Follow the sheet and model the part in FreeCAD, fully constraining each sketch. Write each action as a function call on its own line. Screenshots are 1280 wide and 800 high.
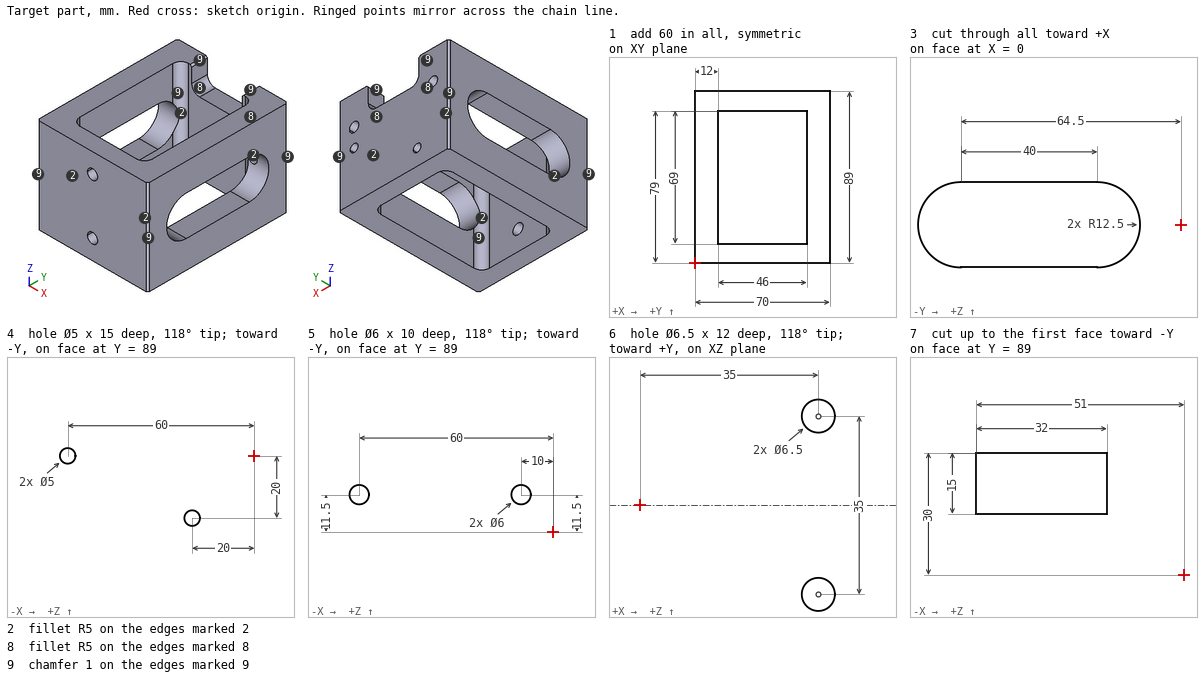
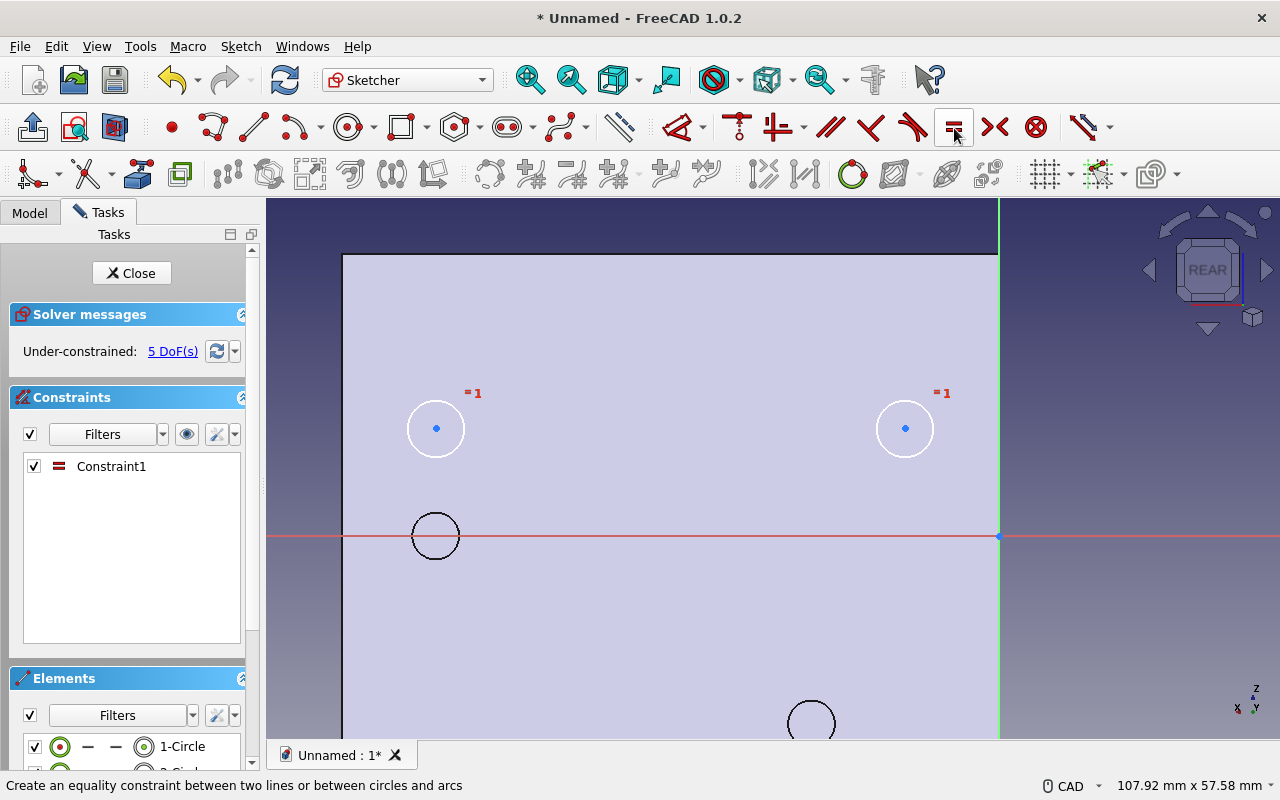
click(925, 409)
click(948, 386)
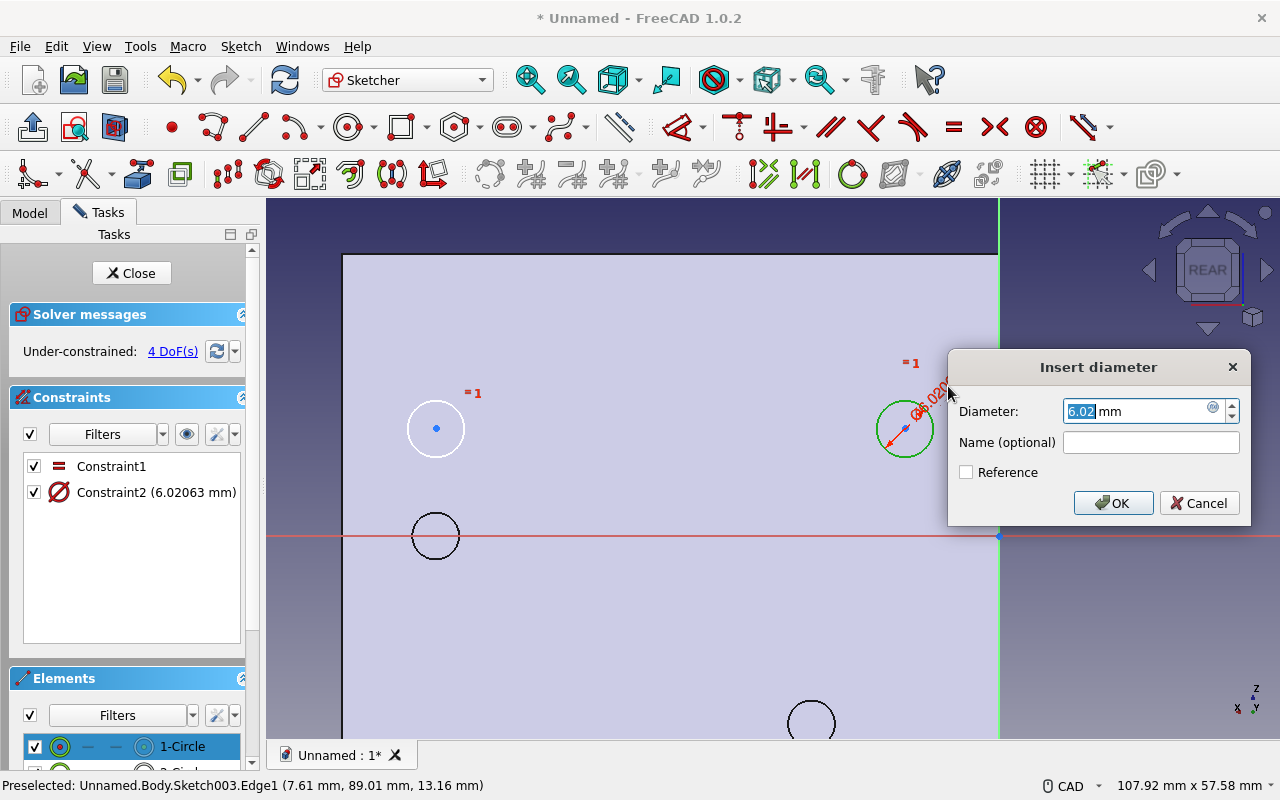
text(6)
key(Return)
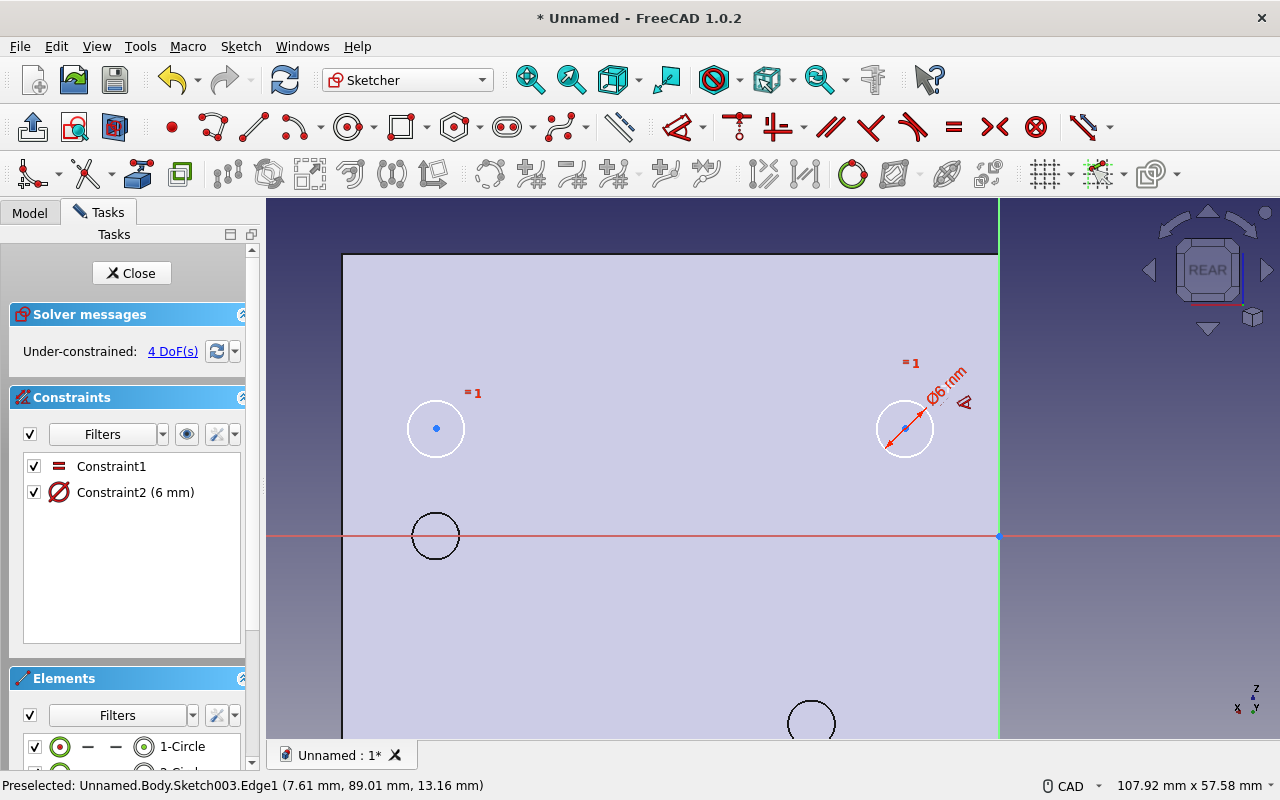
click(905, 429)
click(952, 570)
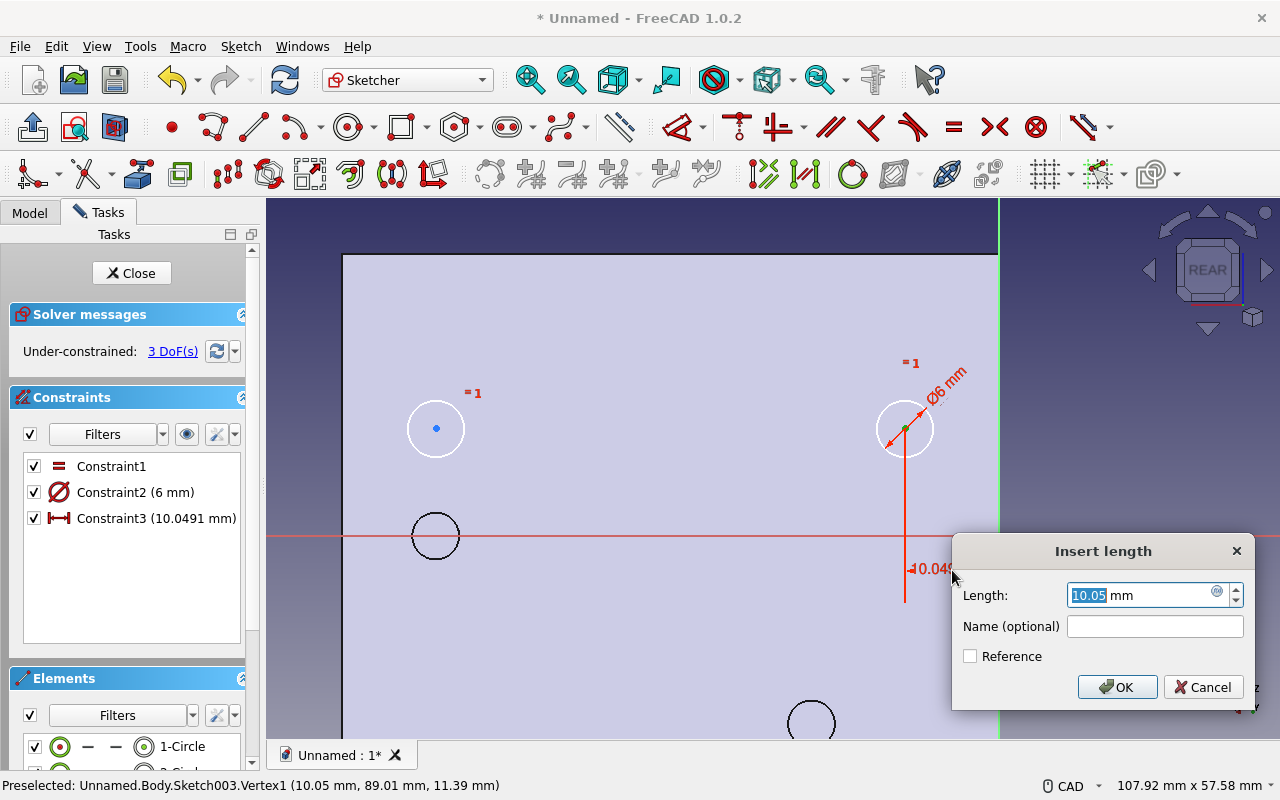
text(10)
key(Return)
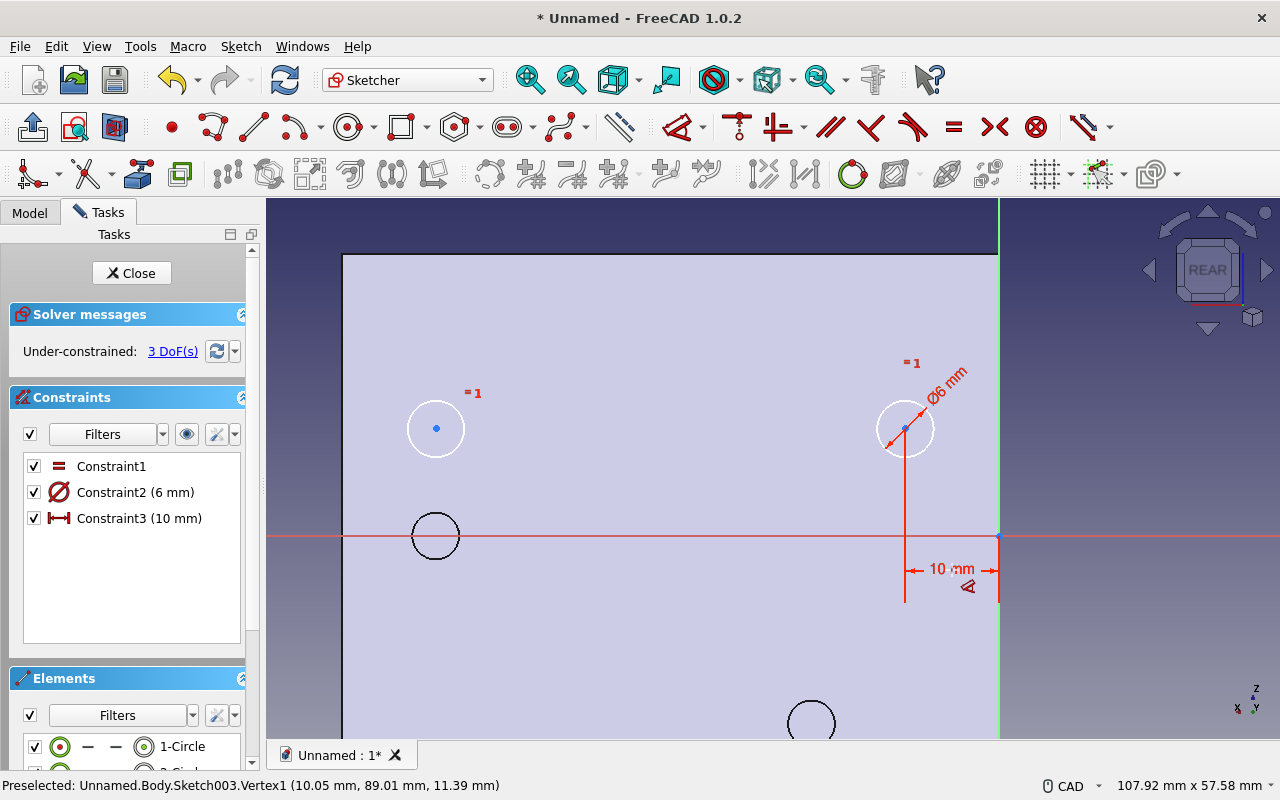
click(436, 429)
click(718, 570)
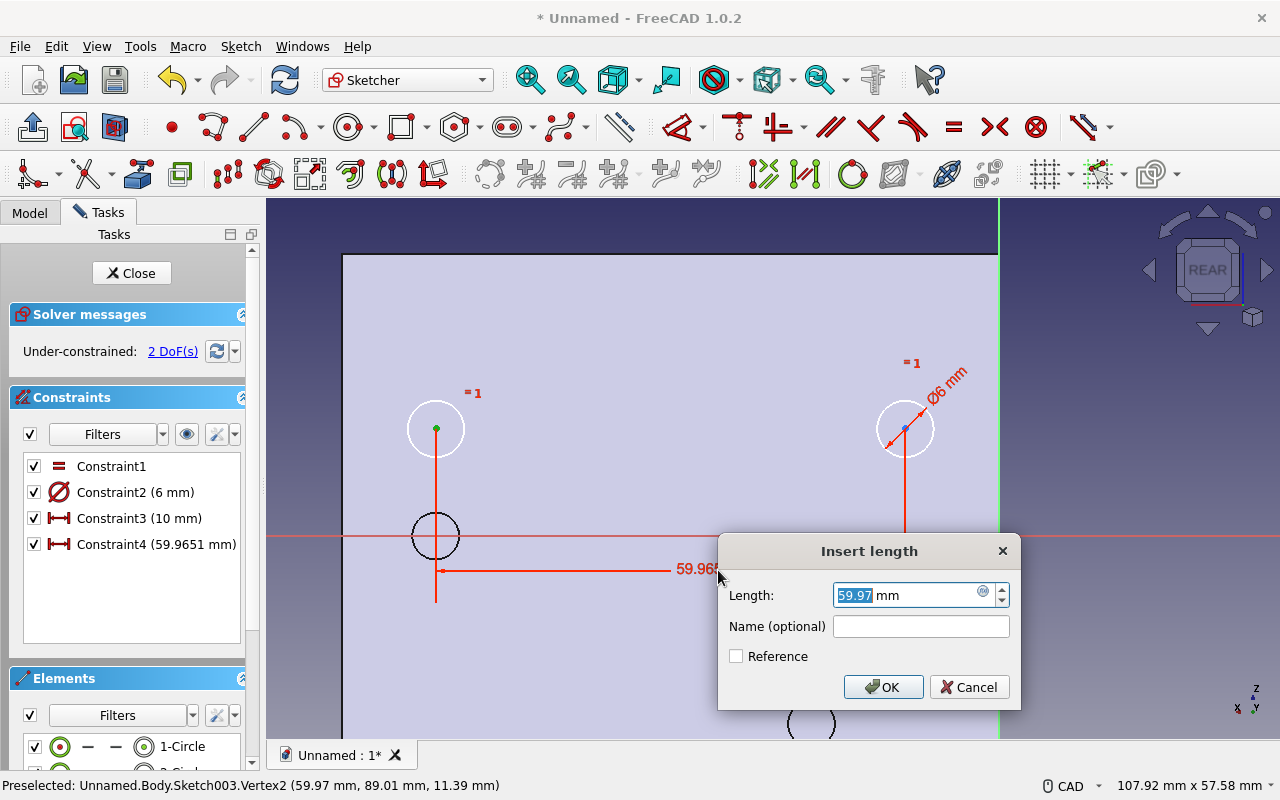
text(60)
key(Return)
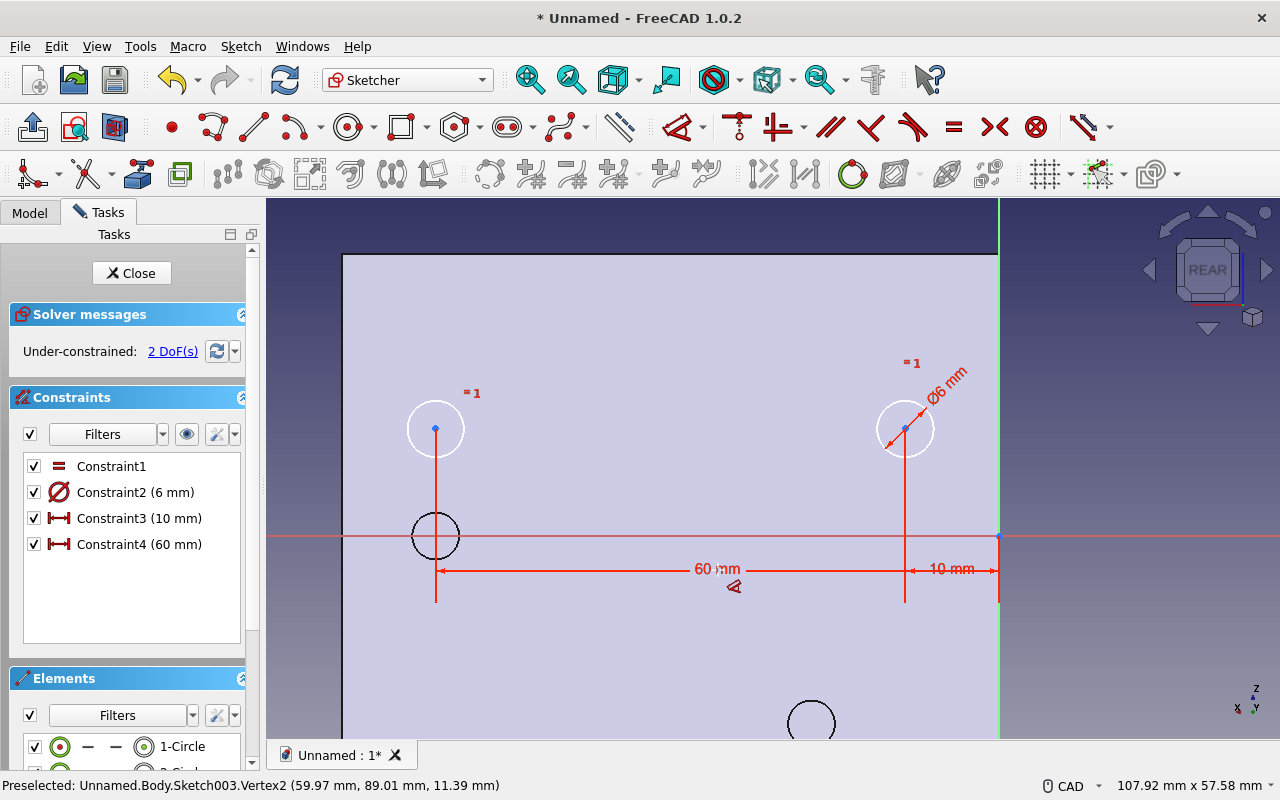
click(905, 429)
click(1033, 483)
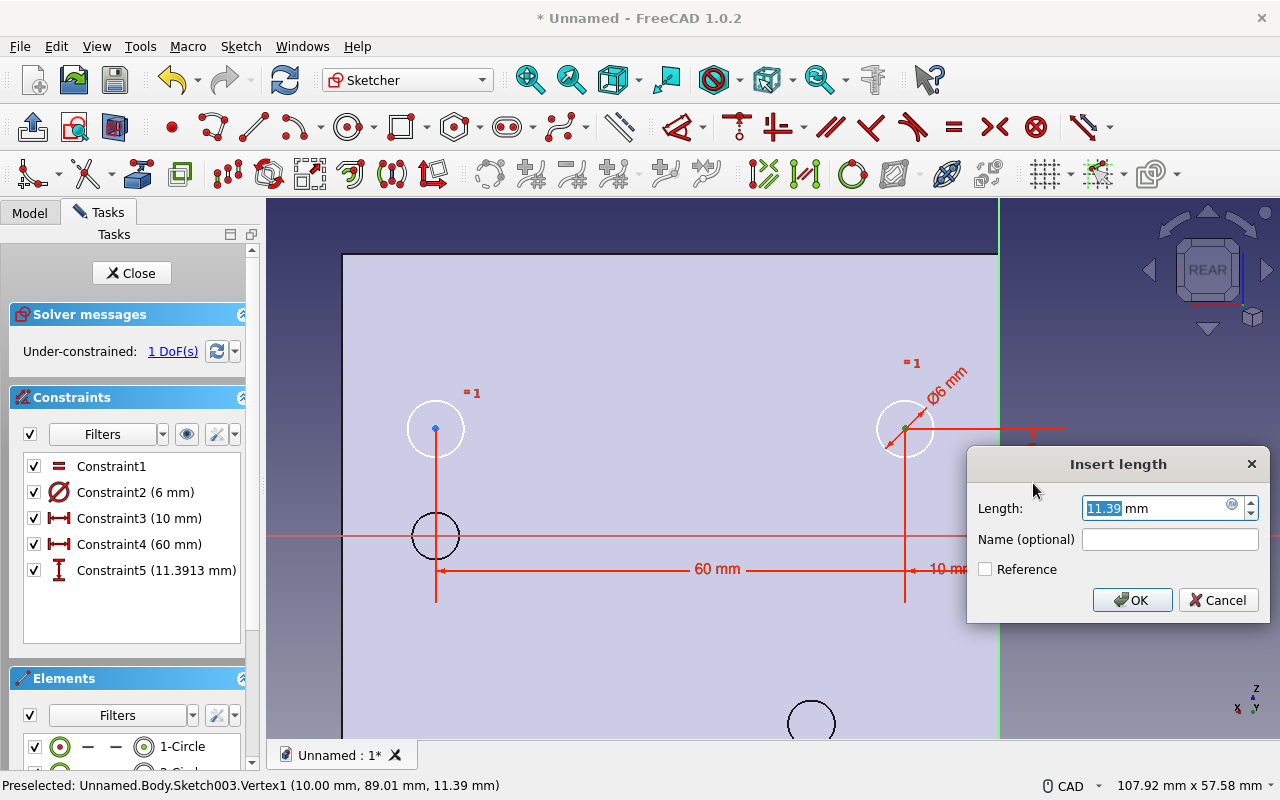
text(11.5)
key(Return)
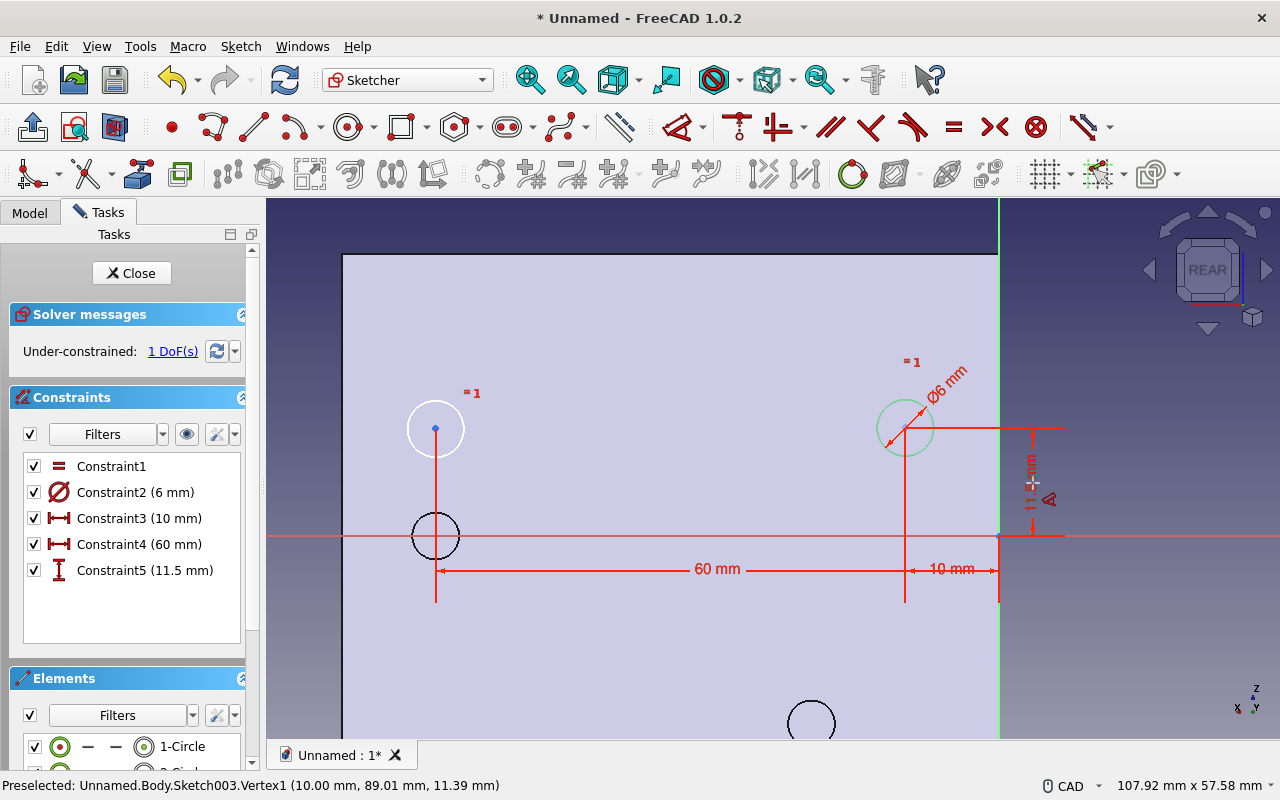
click(436, 429)
click(1033, 458)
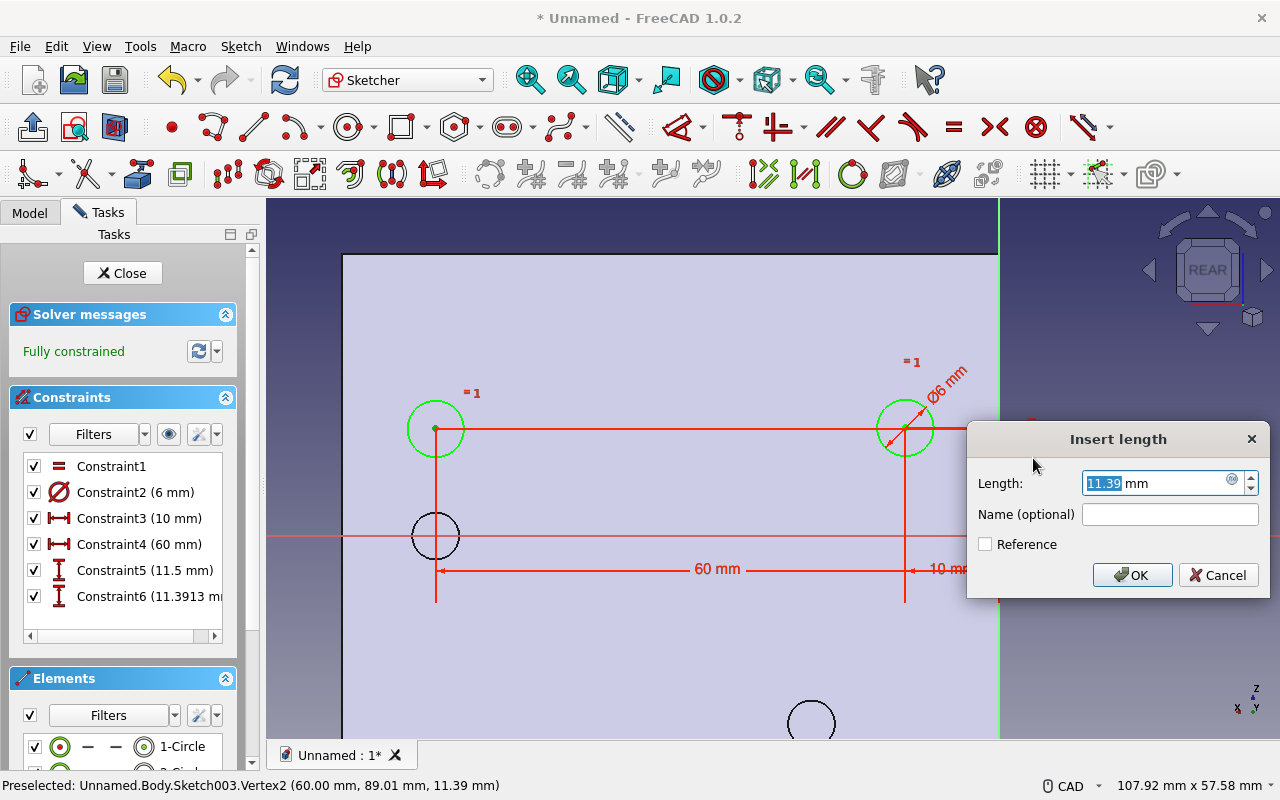
text(11.5)
key(Return)
key(Escape)